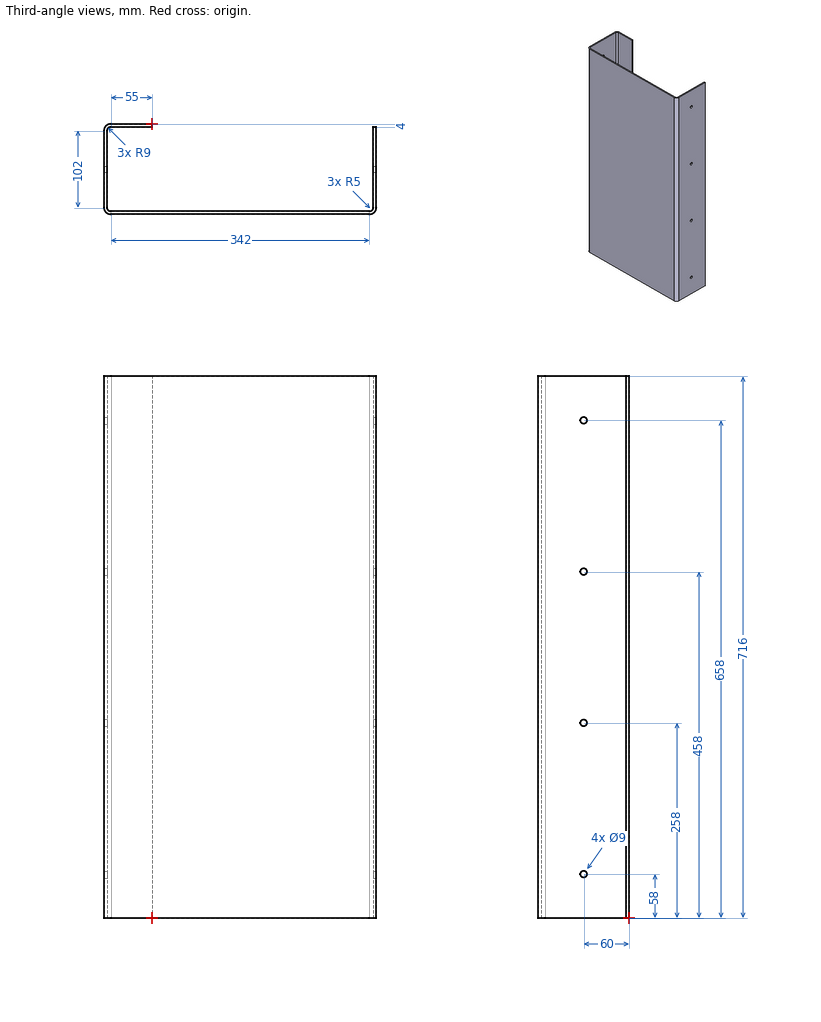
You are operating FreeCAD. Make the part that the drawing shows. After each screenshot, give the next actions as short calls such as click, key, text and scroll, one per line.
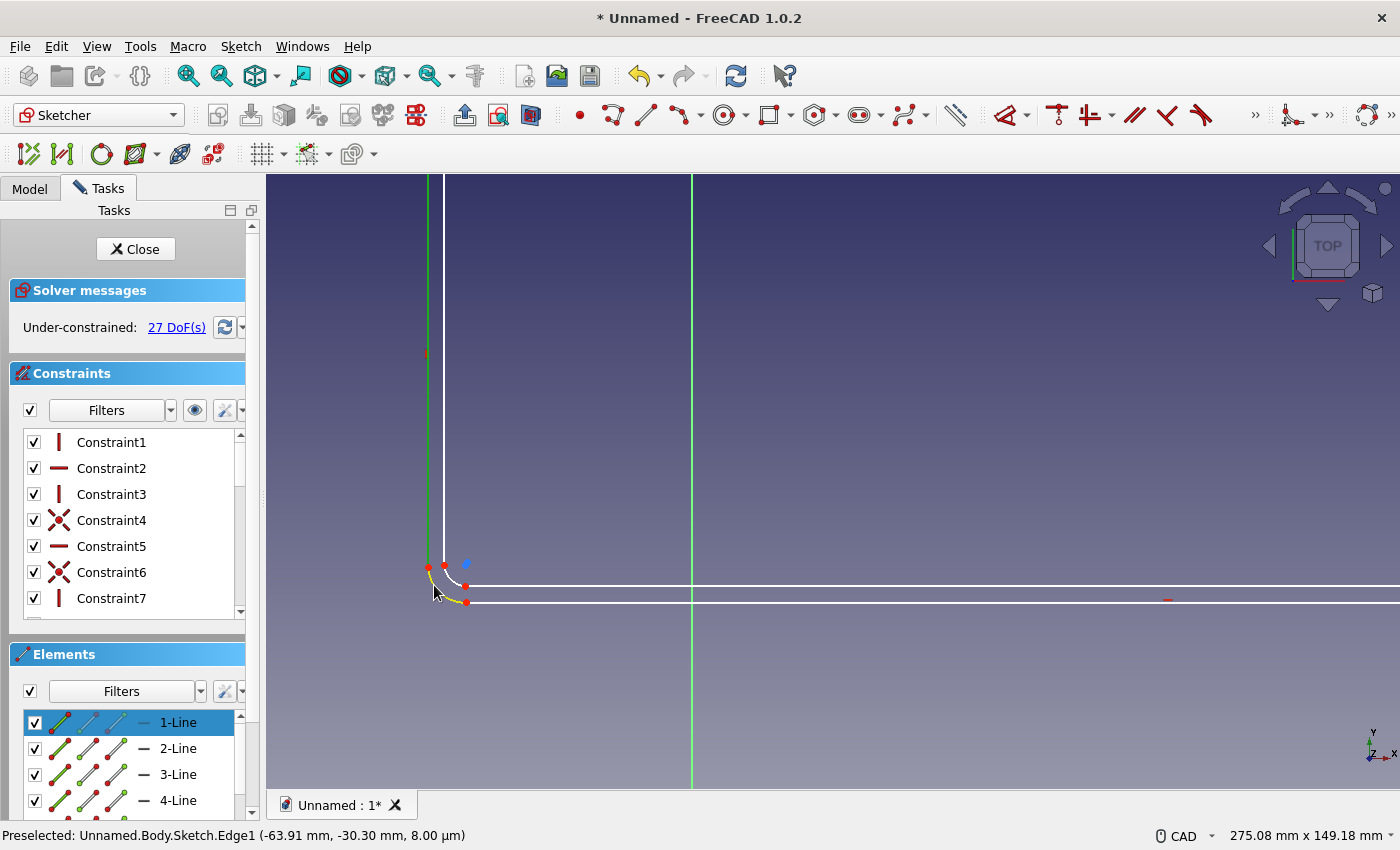
click(433, 584)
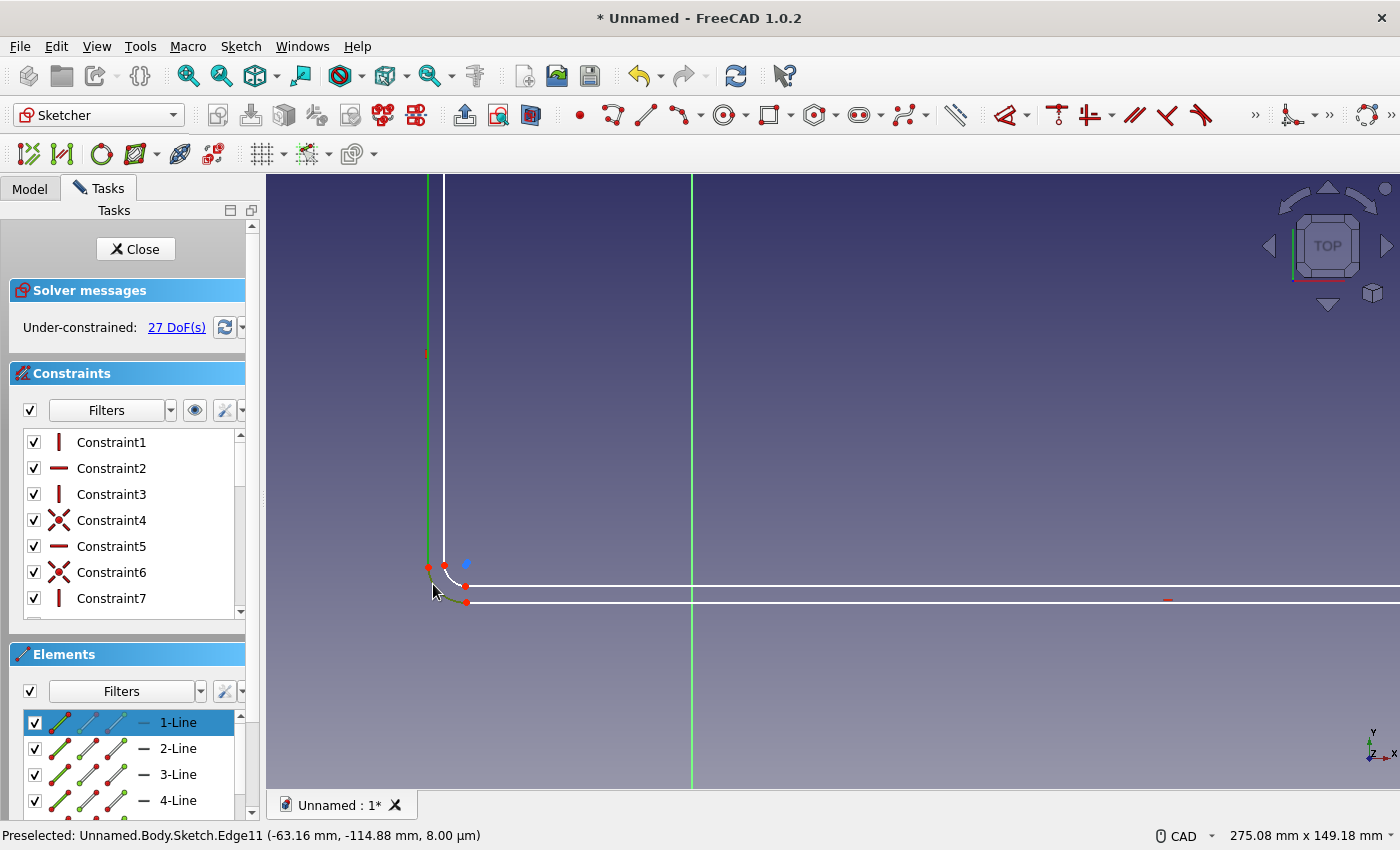
click(1201, 116)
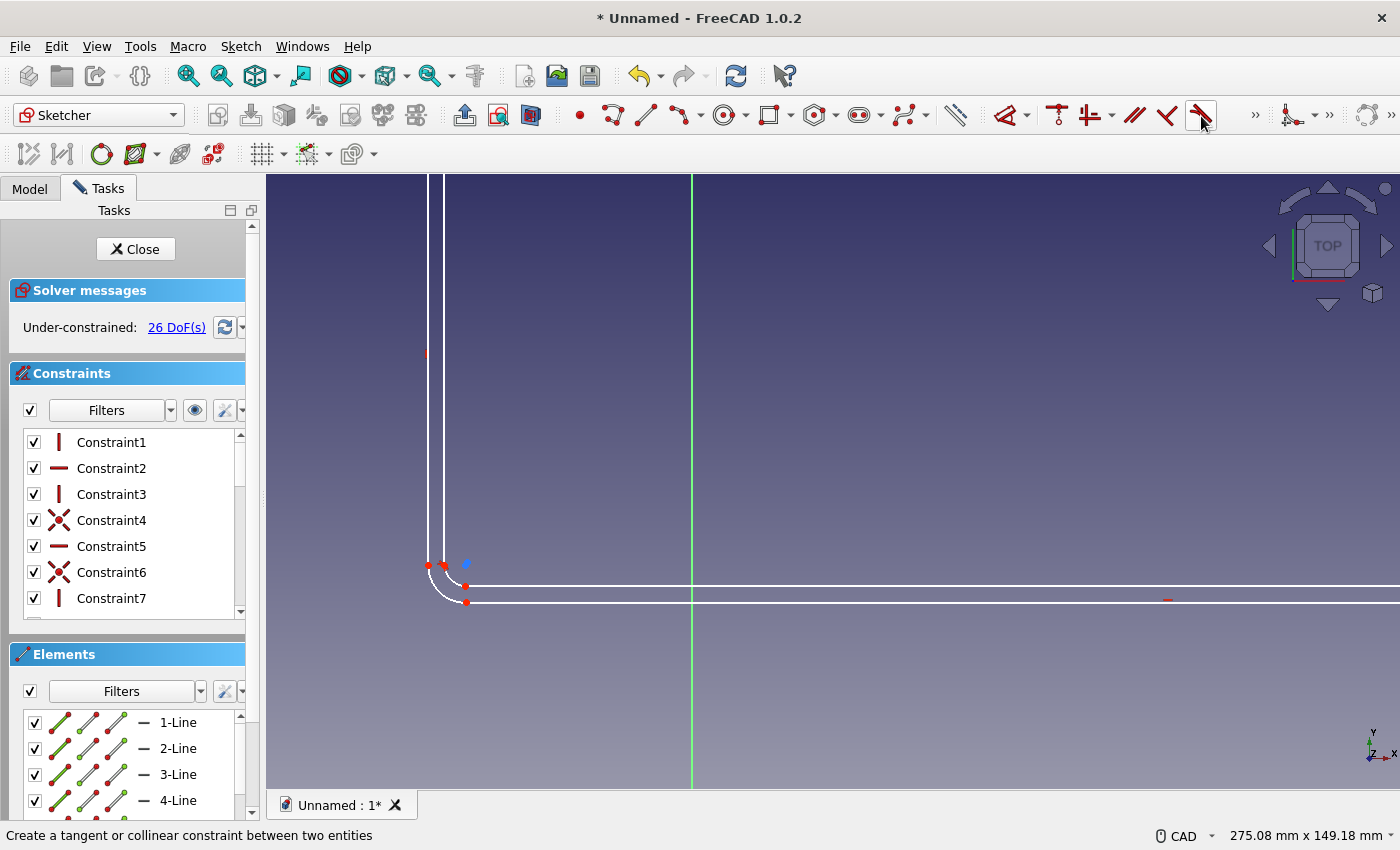
click(428, 272)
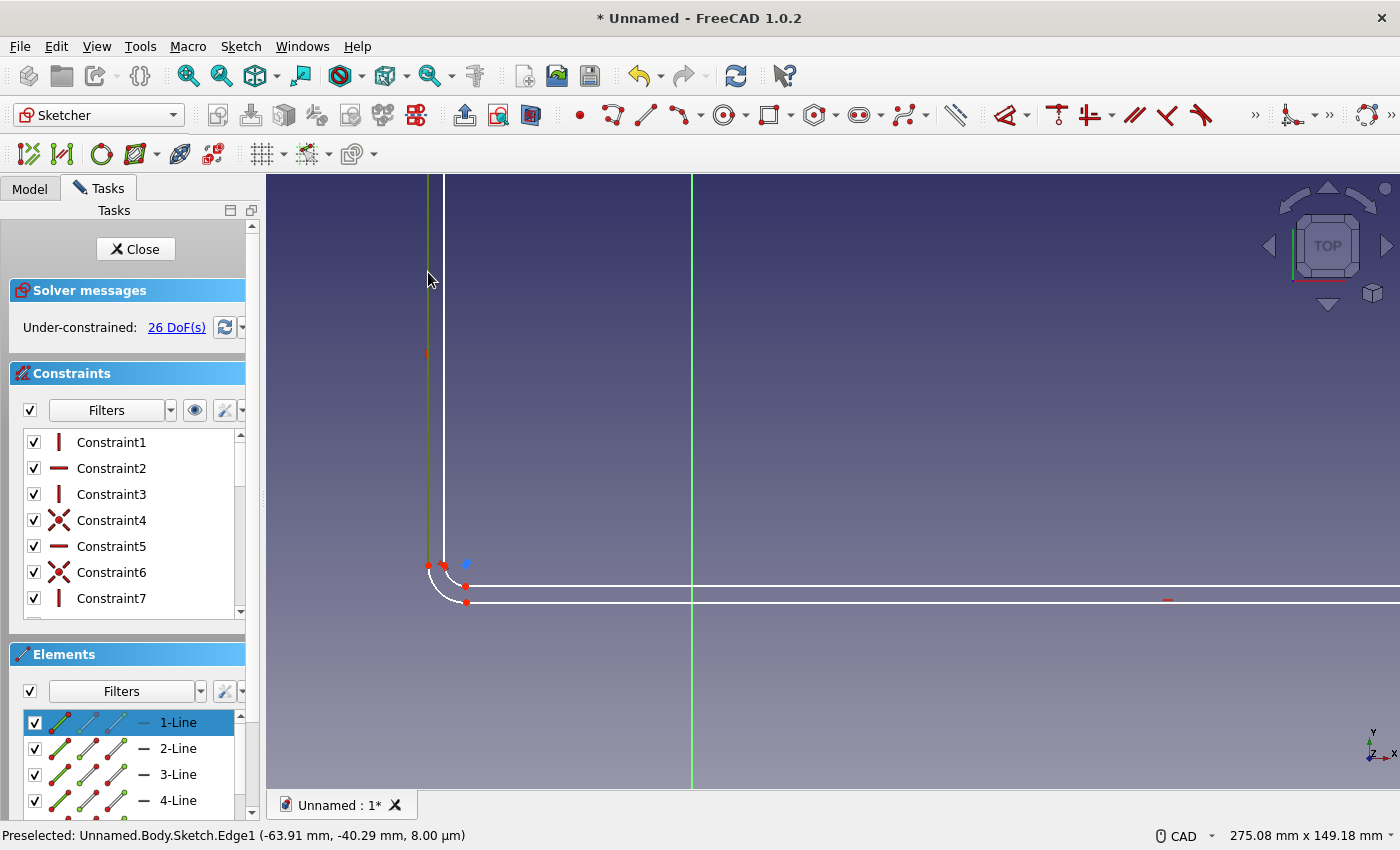
scroll(434, 585, down, 4)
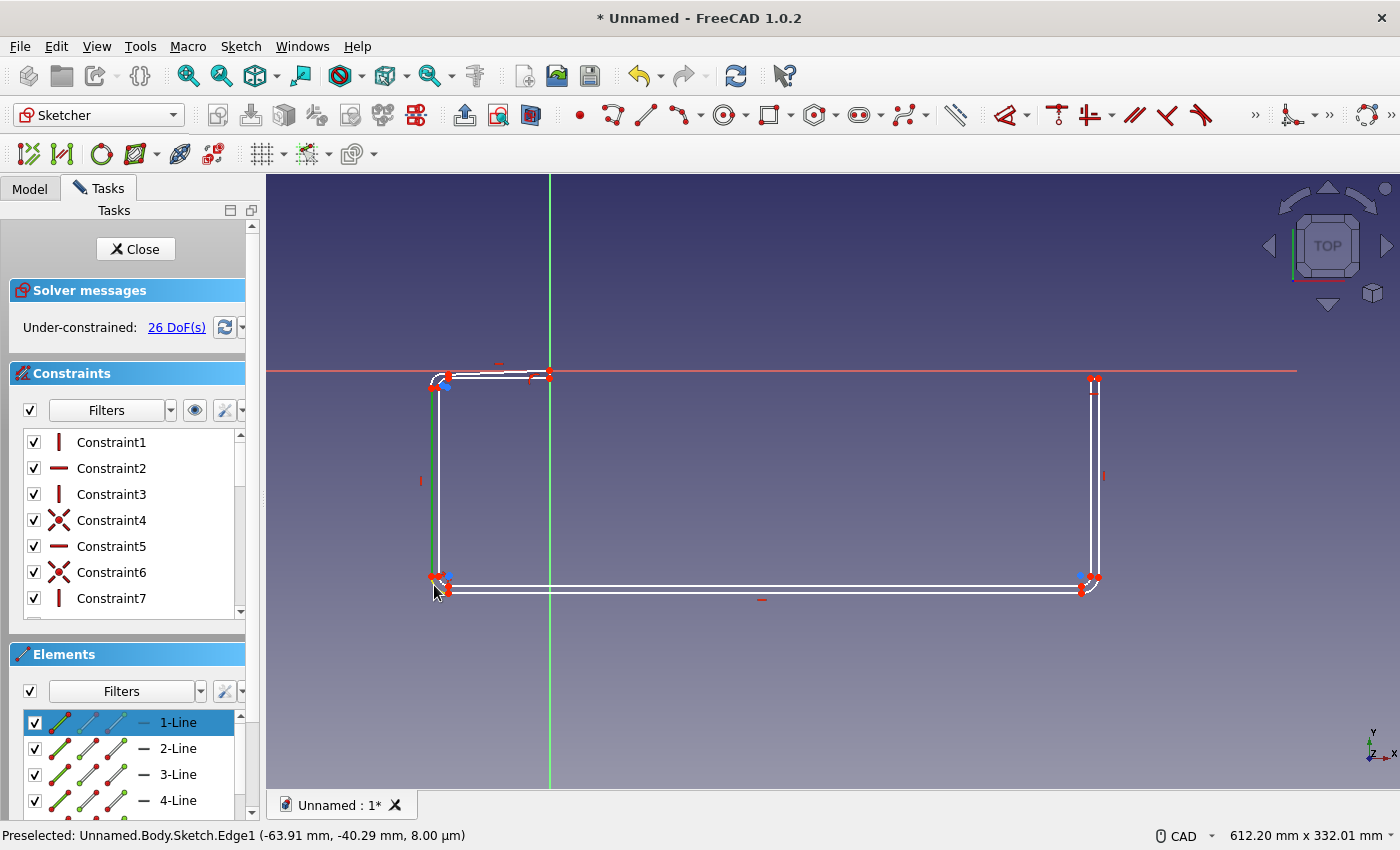
scroll(432, 380, up, 3)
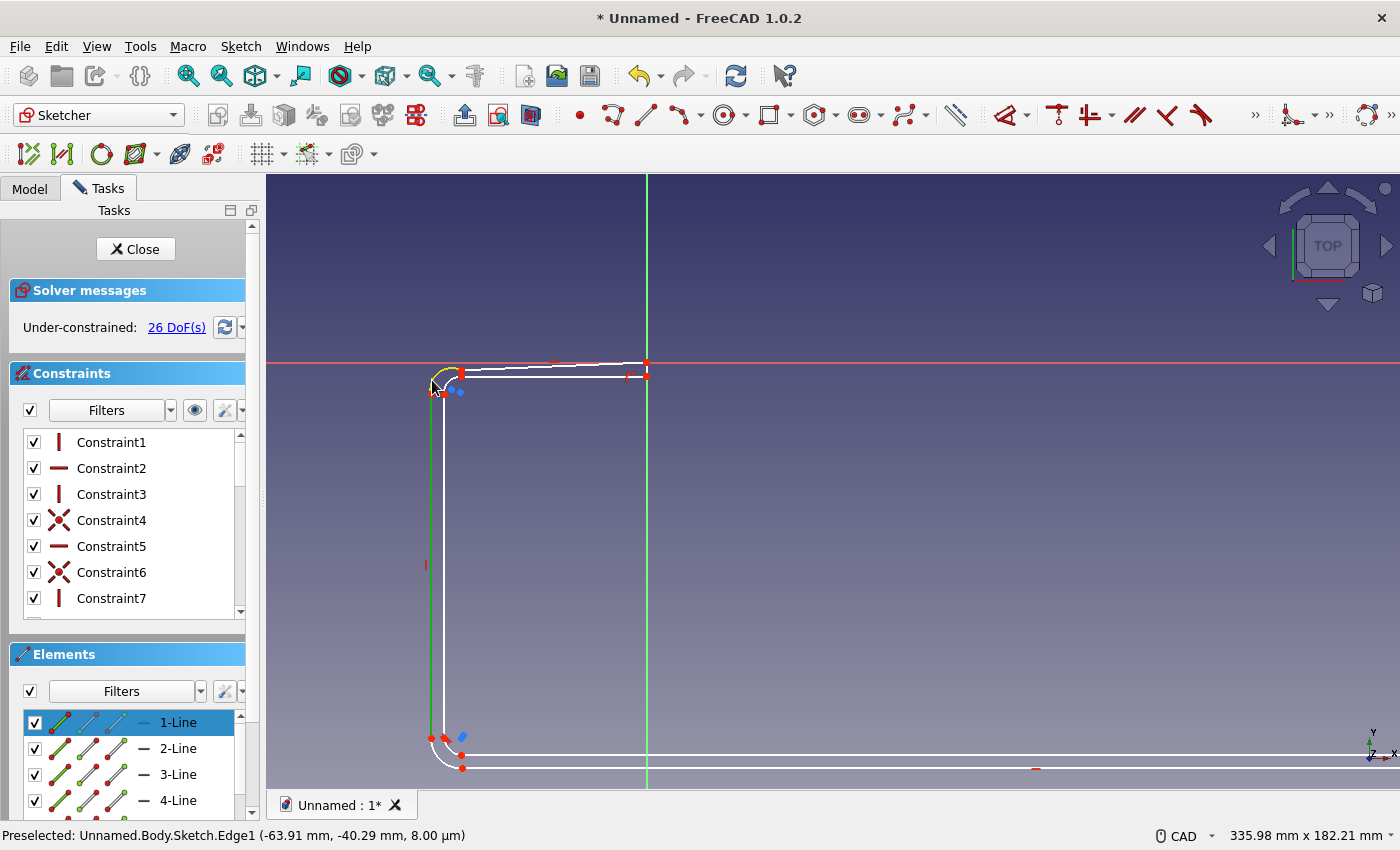
click(432, 381)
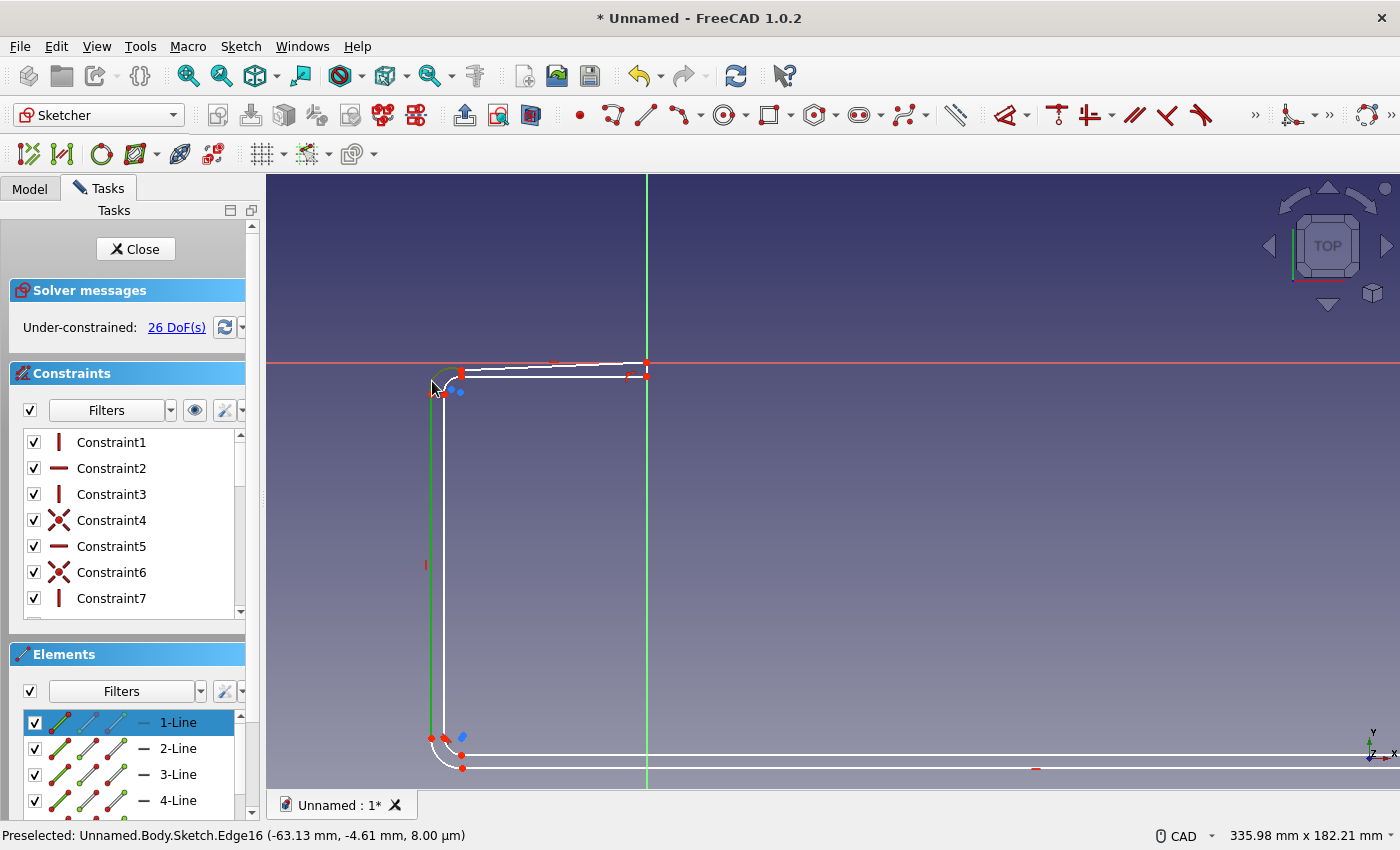
click(1201, 116)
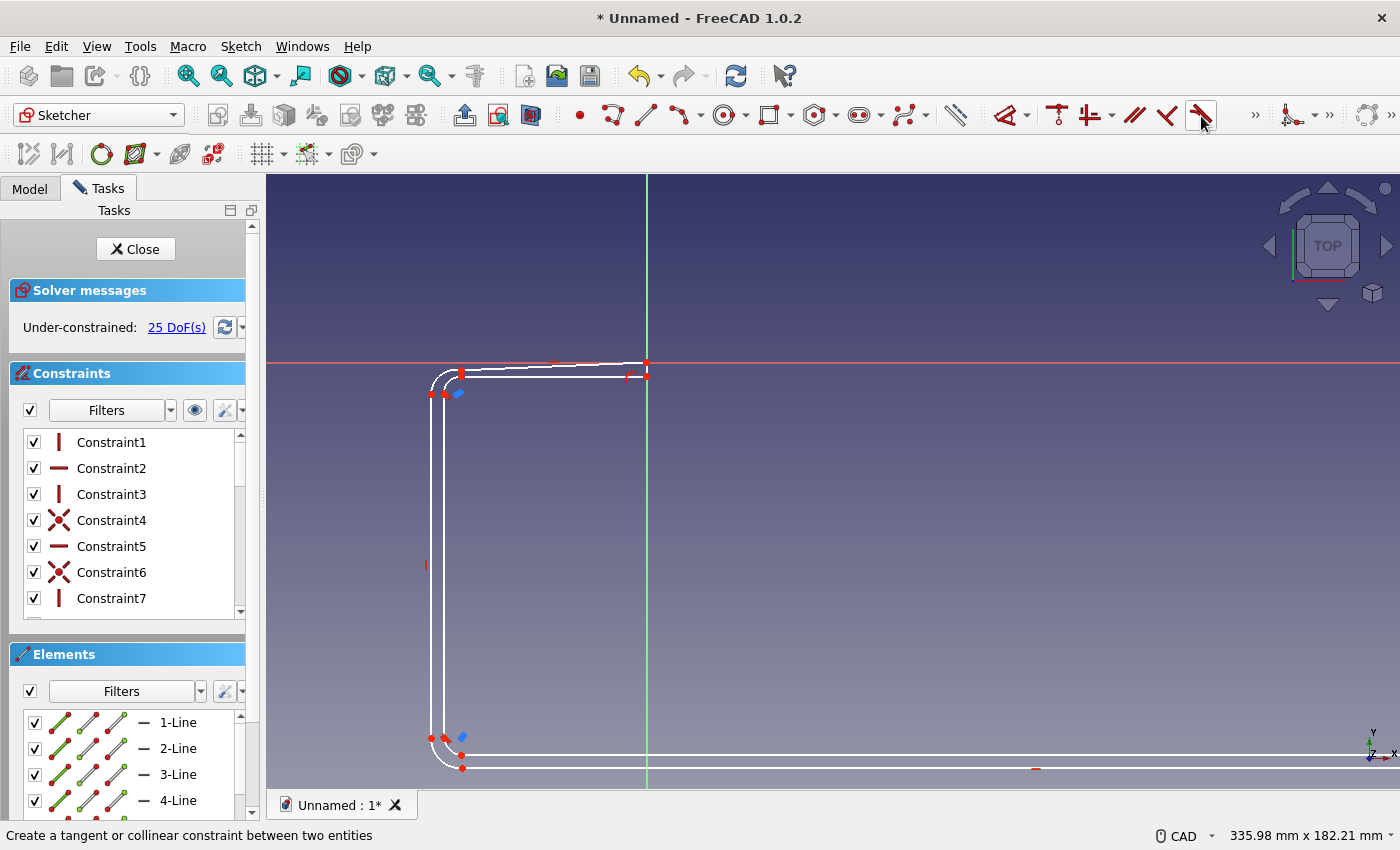
scroll(431, 380, down, 3)